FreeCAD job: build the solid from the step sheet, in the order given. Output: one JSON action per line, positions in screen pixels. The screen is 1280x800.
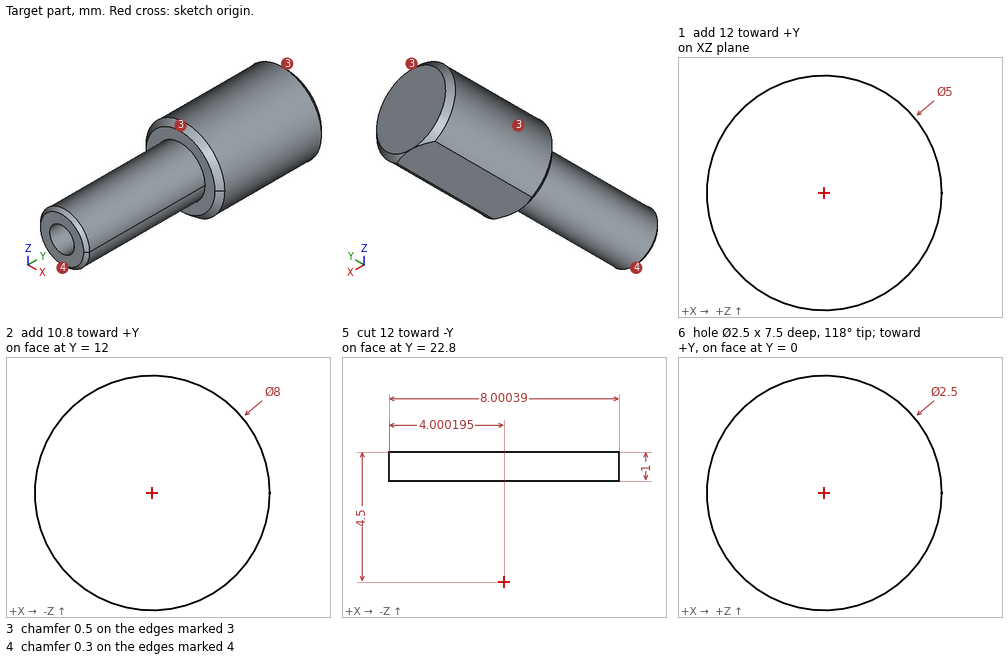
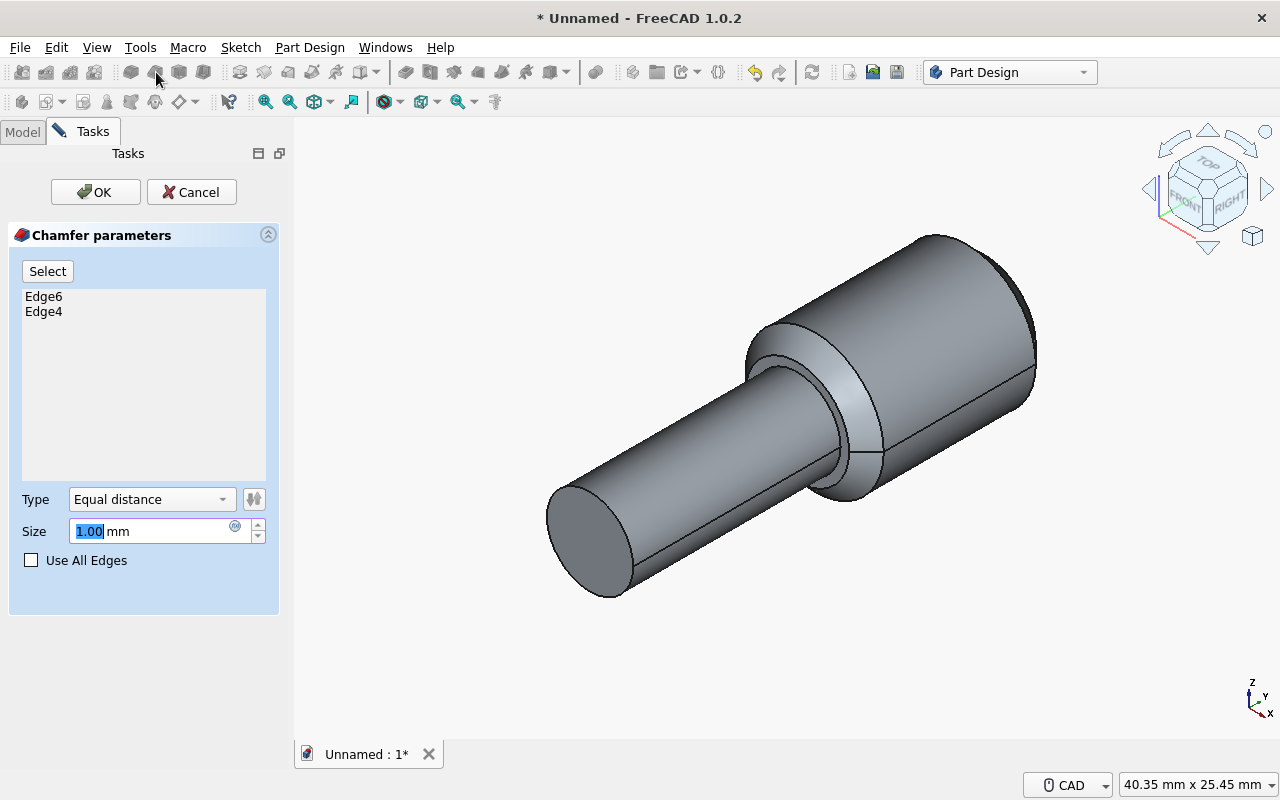
{"action": "type", "text": "0.5"}
{"action": "key", "text": "Tab"}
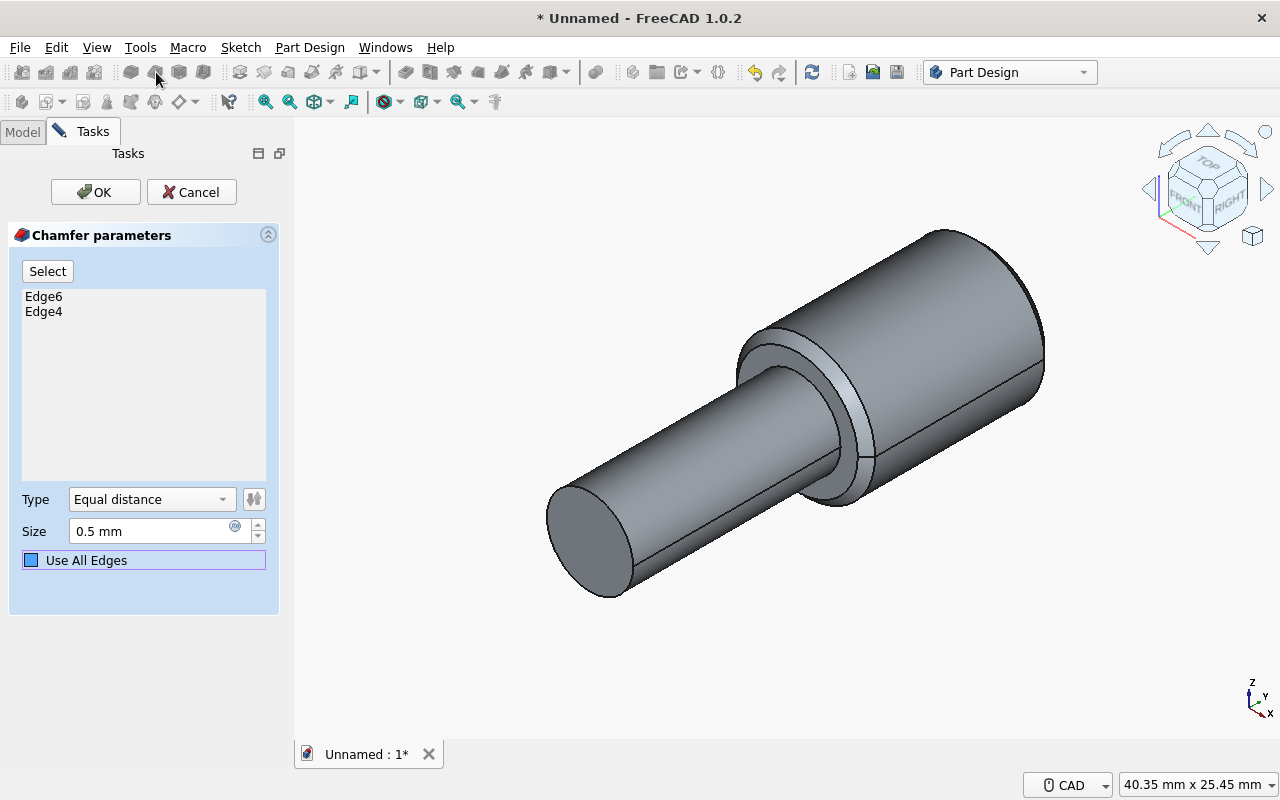
{"action": "left_click", "coordinate": [96, 192]}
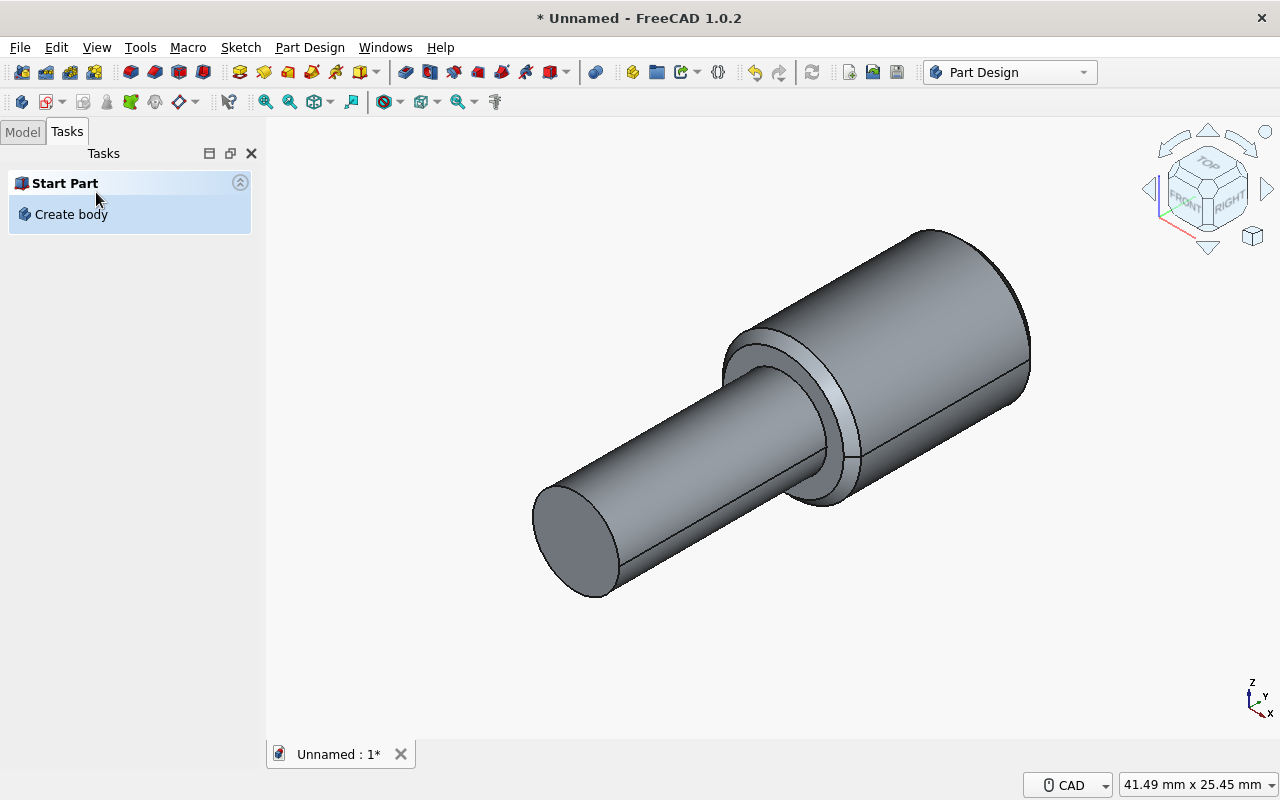
{"action": "left_click", "coordinate": [563, 486]}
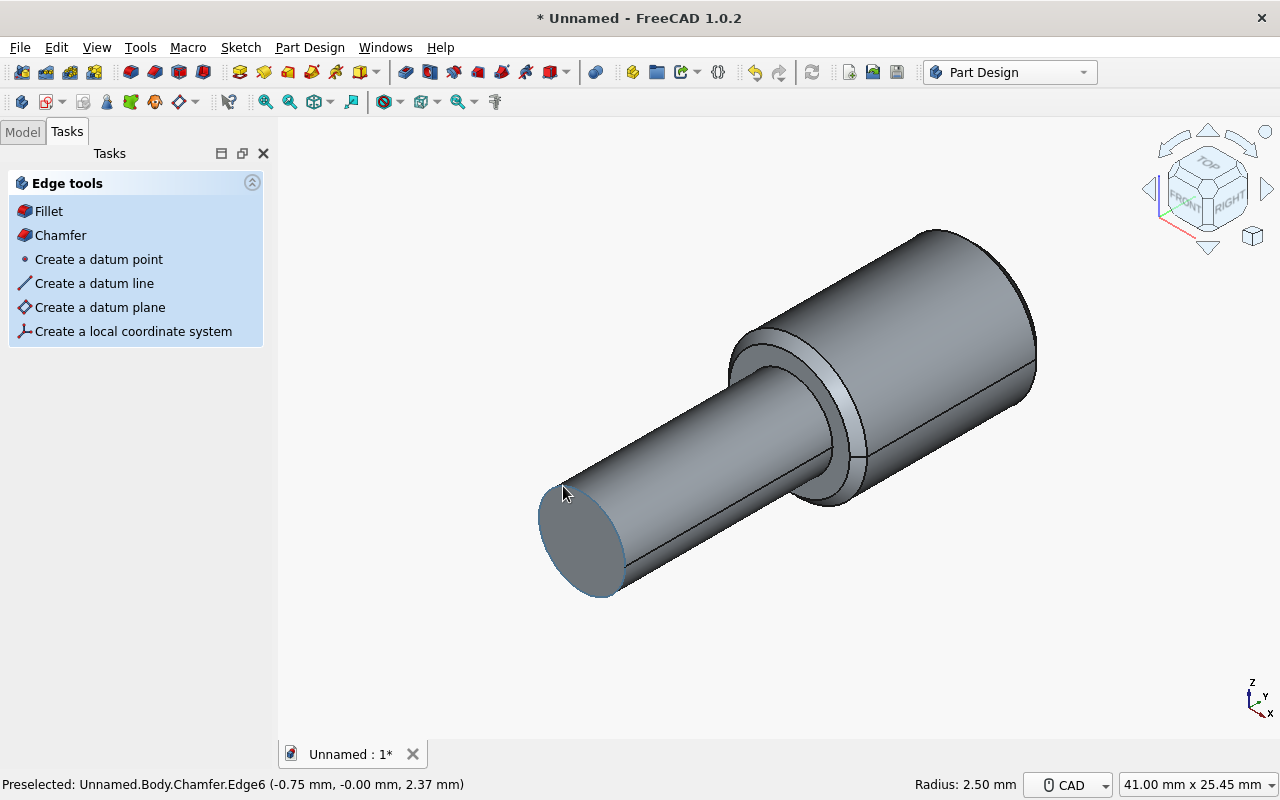
{"action": "left_click", "coordinate": [156, 72]}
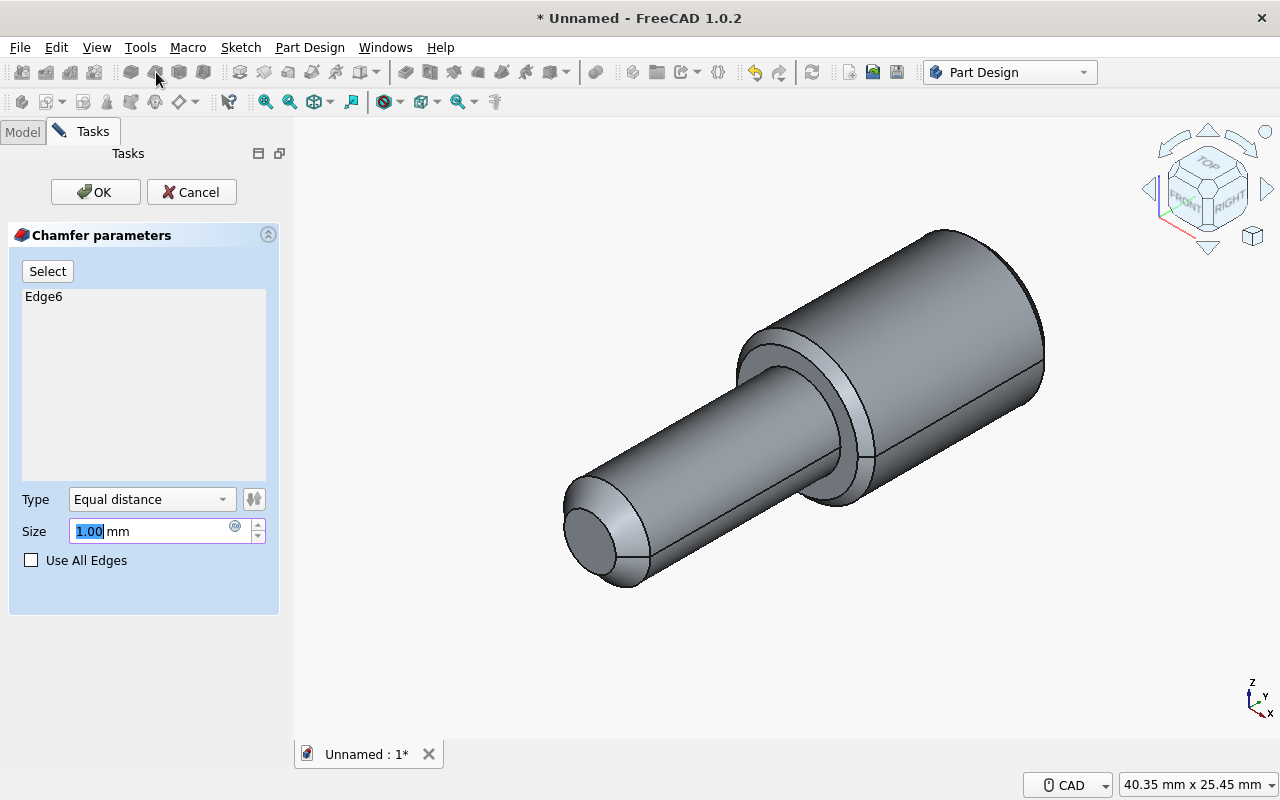
{"action": "type", "text": "0.3"}
{"action": "key", "text": "Tab"}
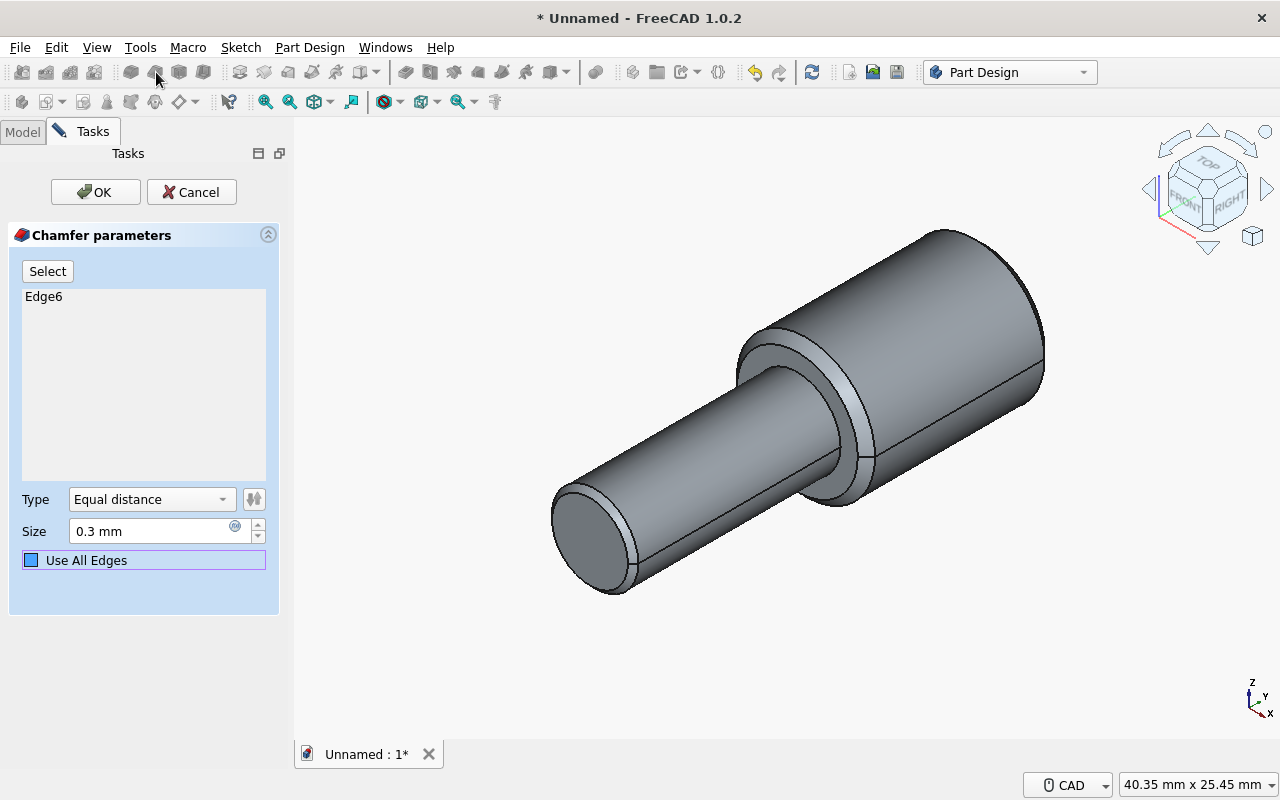
{"action": "left_click", "coordinate": [96, 192]}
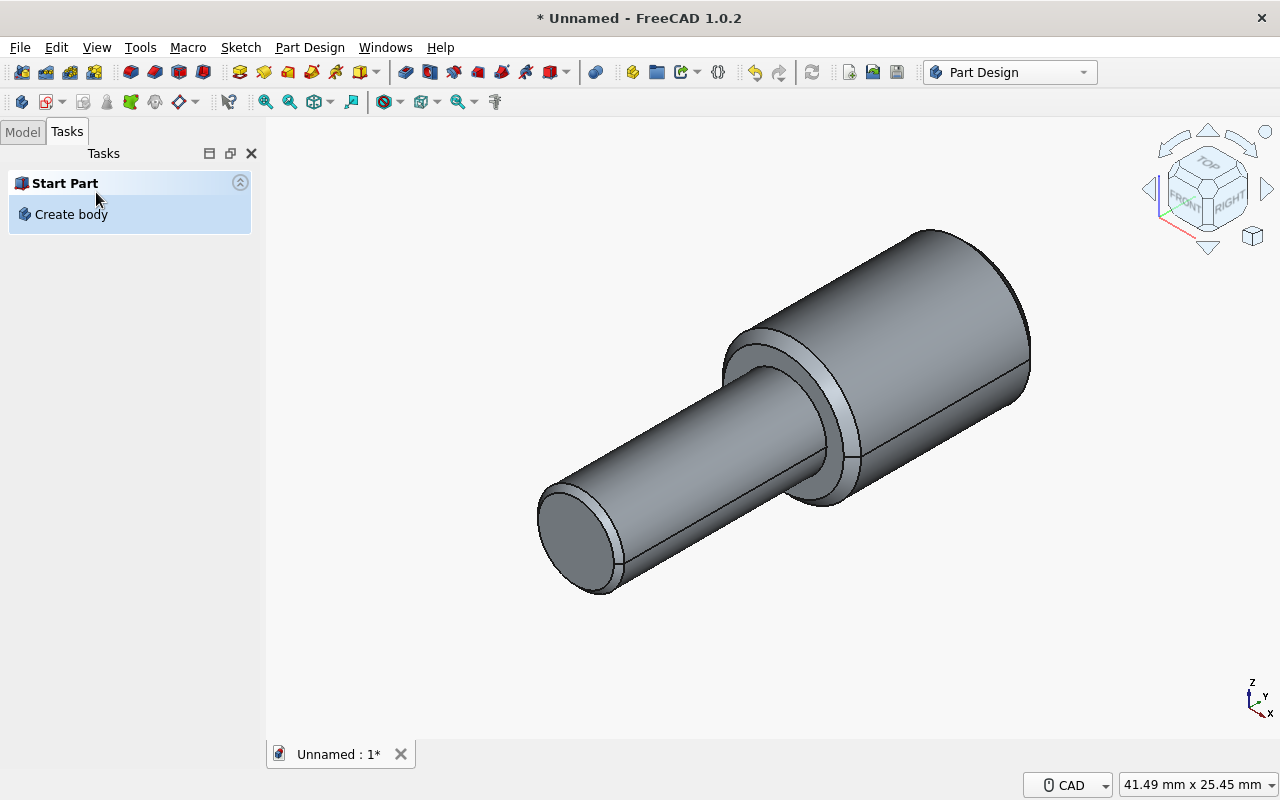
{"action": "key", "text": "4"}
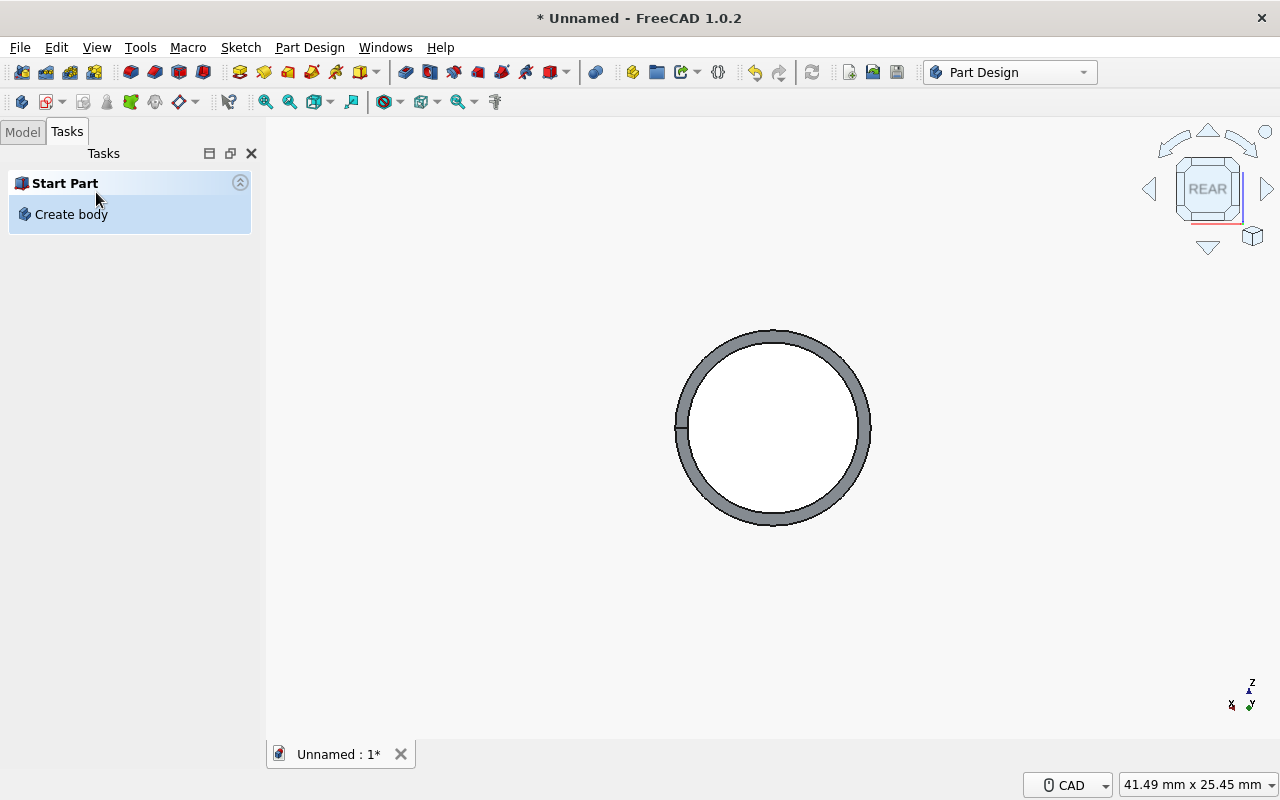
{"action": "key", "text": "v f"}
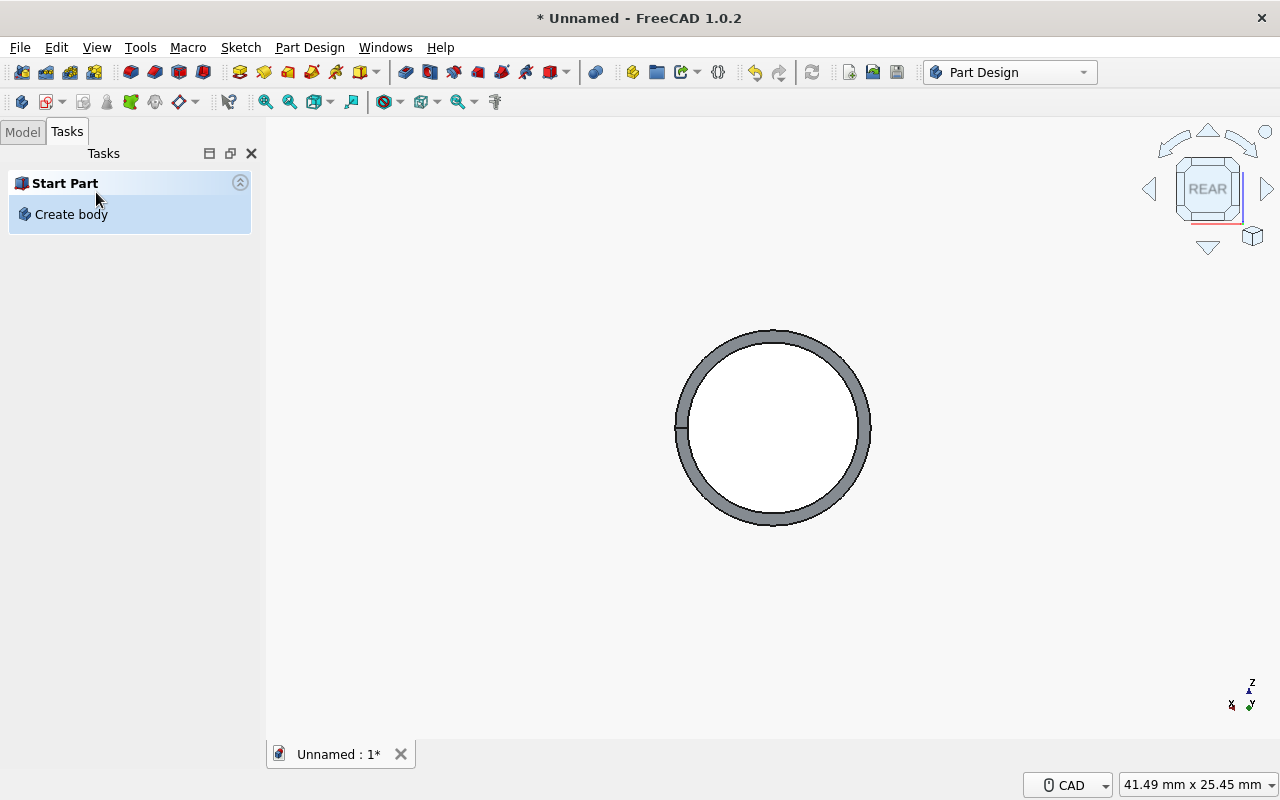
{"action": "left_click", "coordinate": [773, 427]}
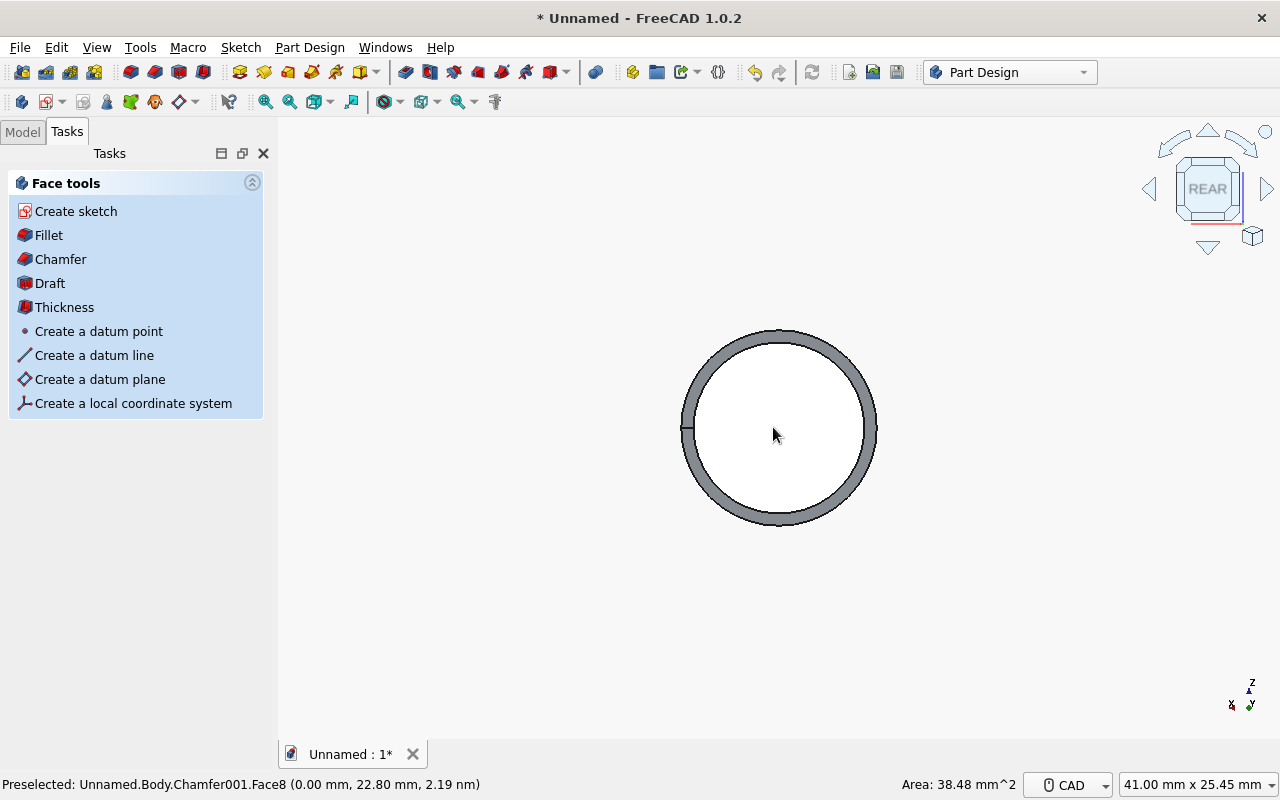
{"action": "left_click", "coordinate": [46, 102]}